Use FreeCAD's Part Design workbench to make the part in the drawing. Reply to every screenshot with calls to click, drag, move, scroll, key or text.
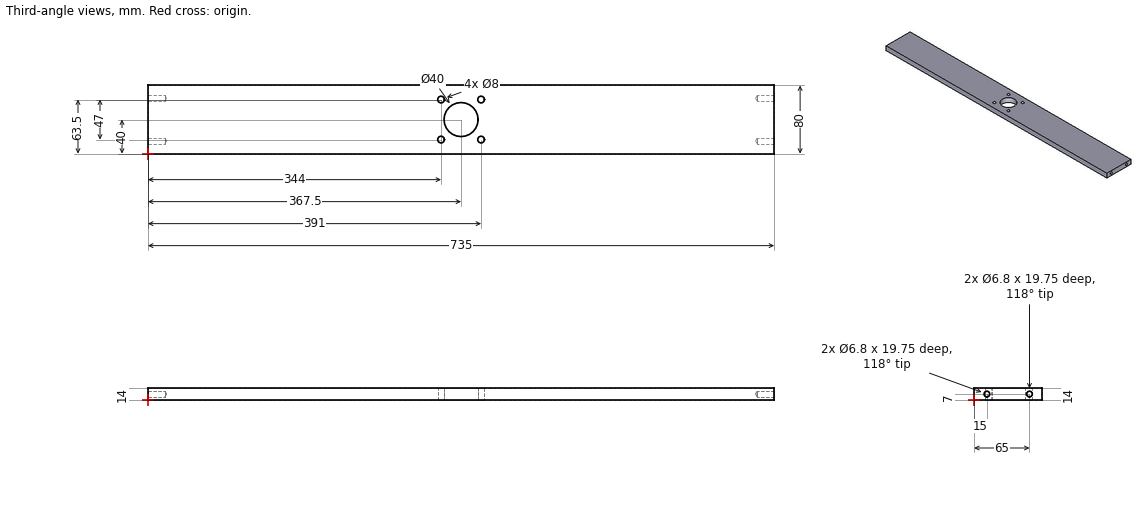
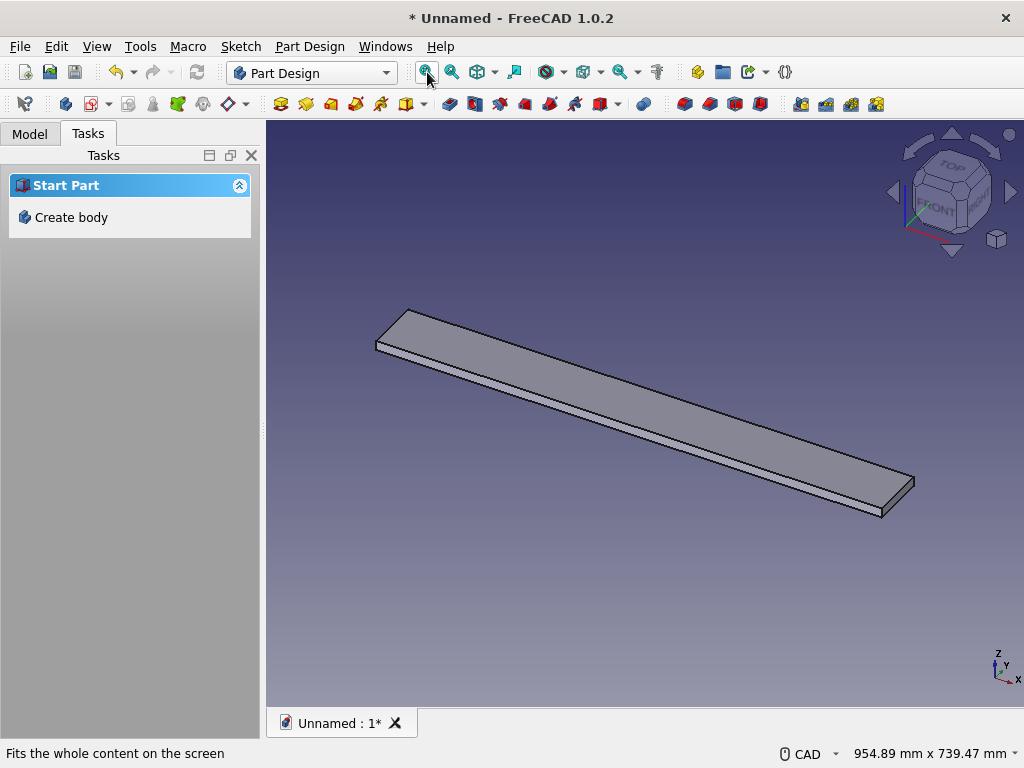
click(862, 480)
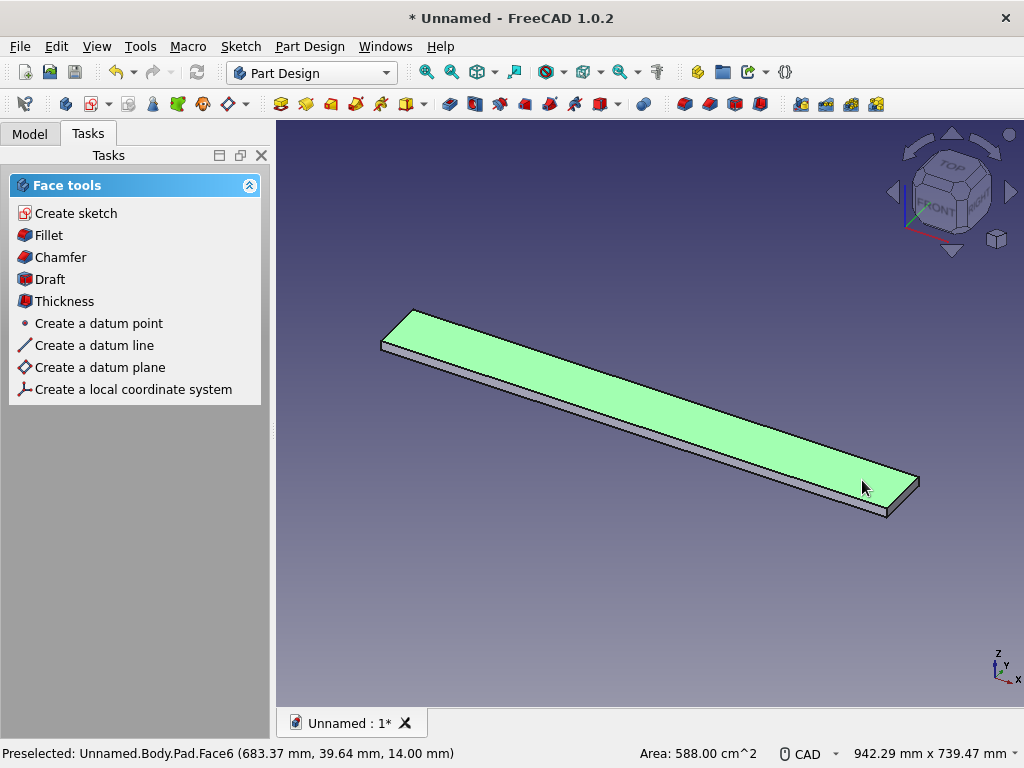
click(90, 104)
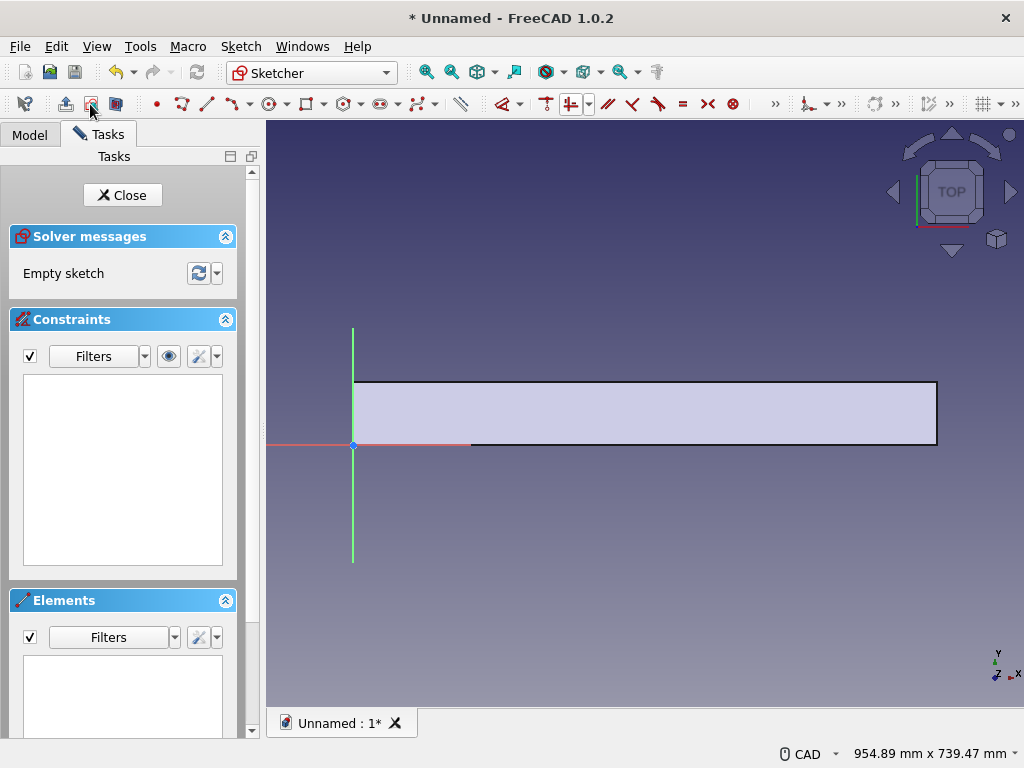
scroll(654, 414, up, 11)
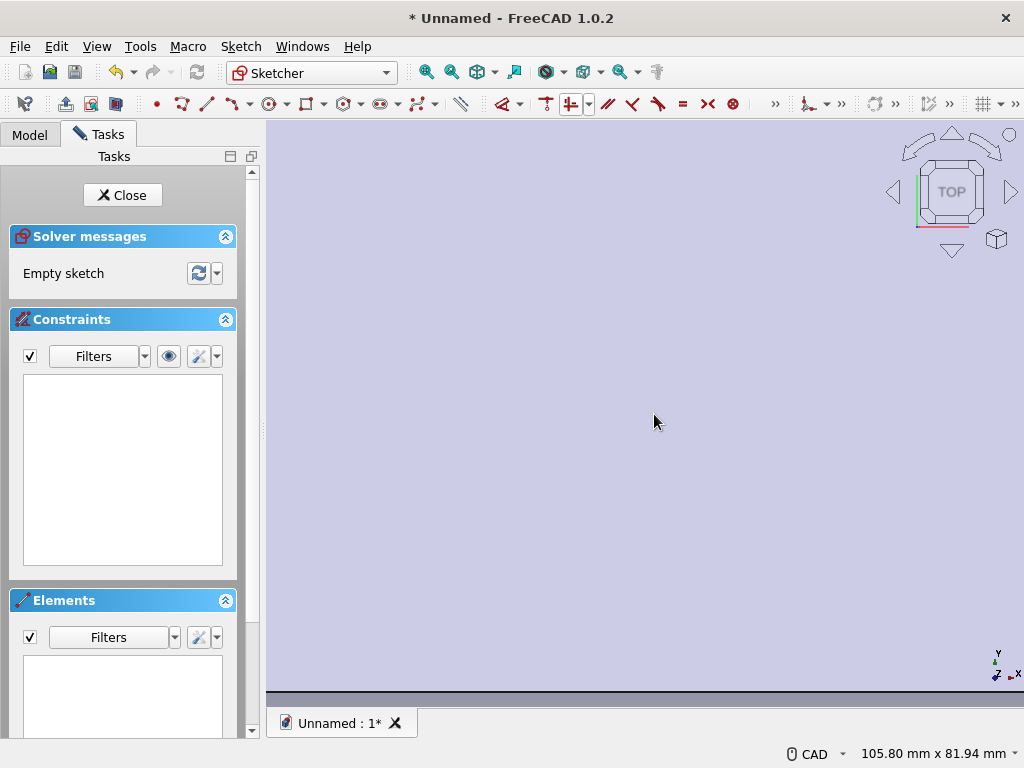
key(g)
key(c)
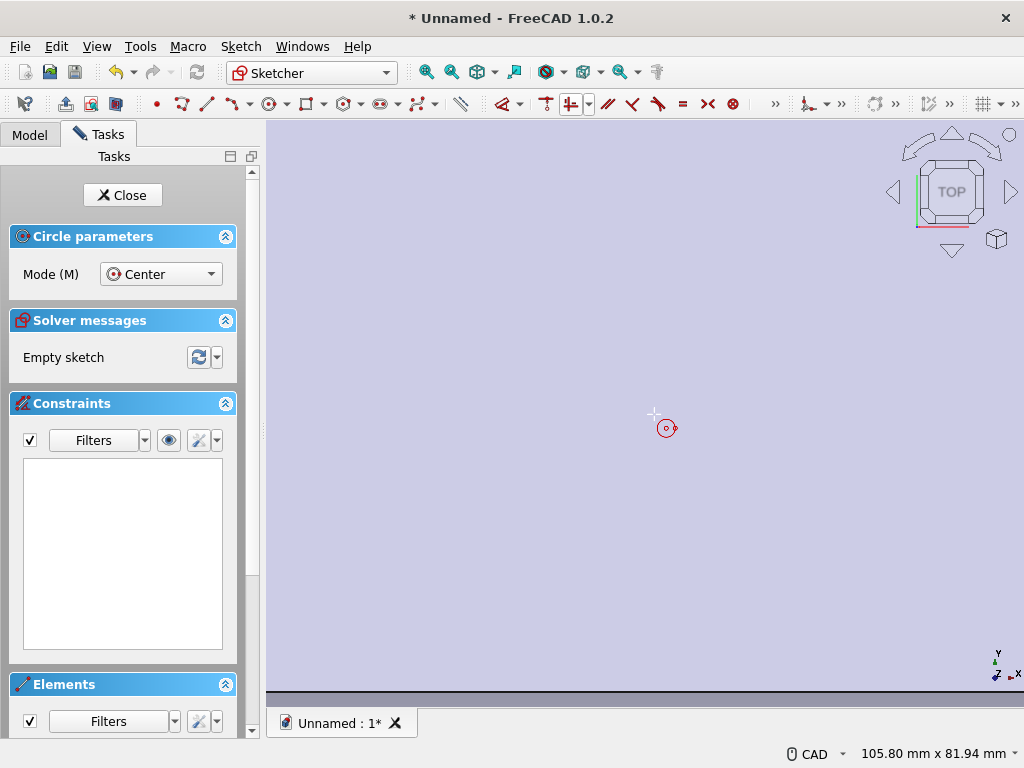
click(400, 237)
move(421, 217)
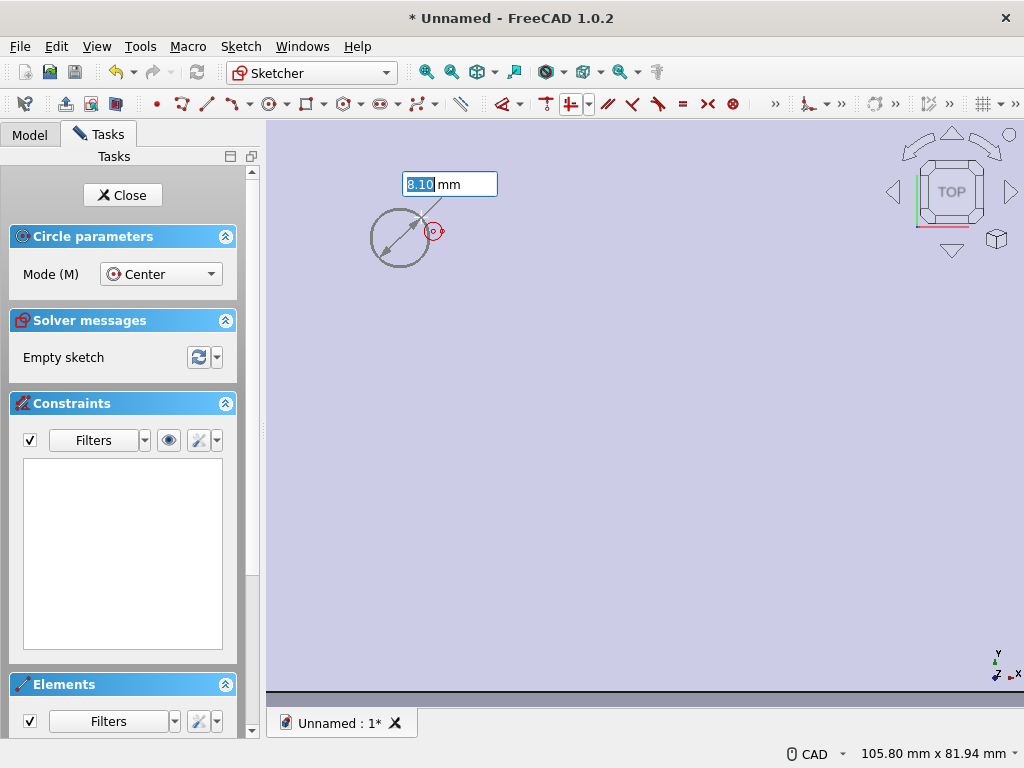
text(8)
key(Return)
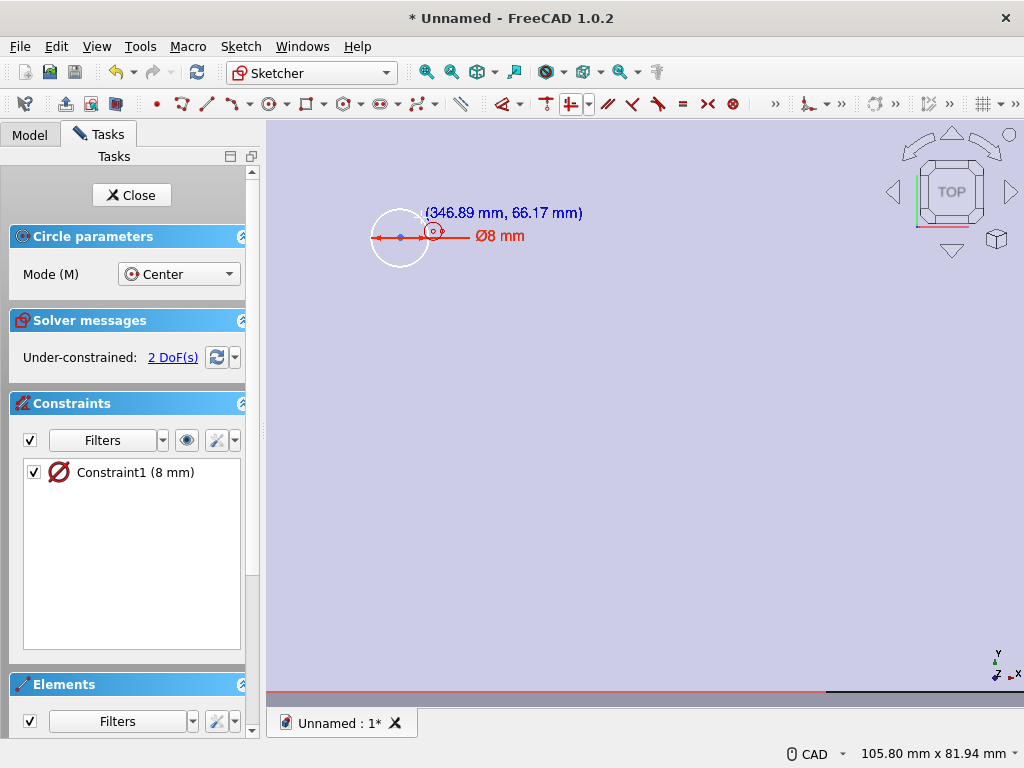
click(400, 574)
move(421, 554)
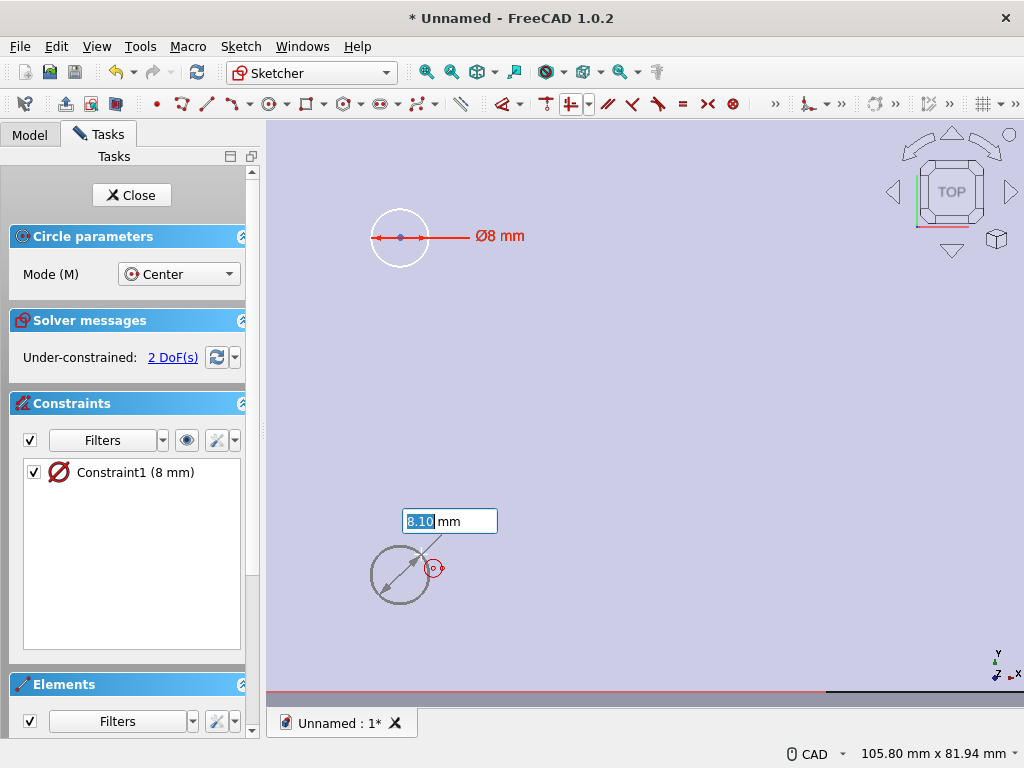
text(8)
key(Return)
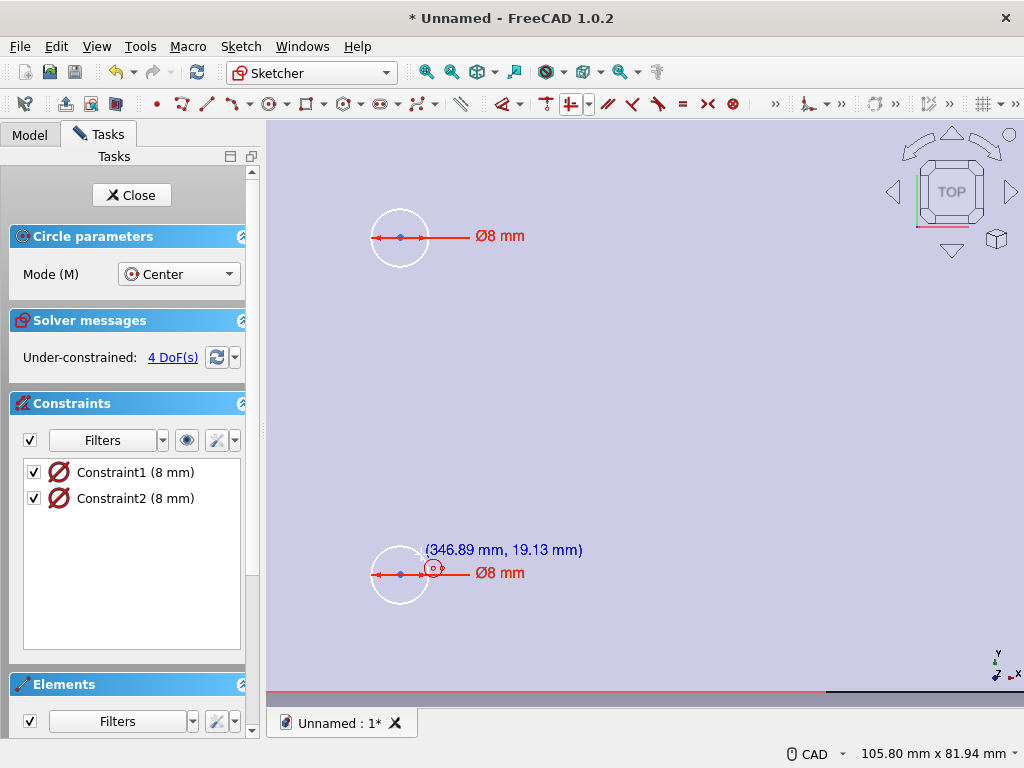
click(737, 574)
move(757, 554)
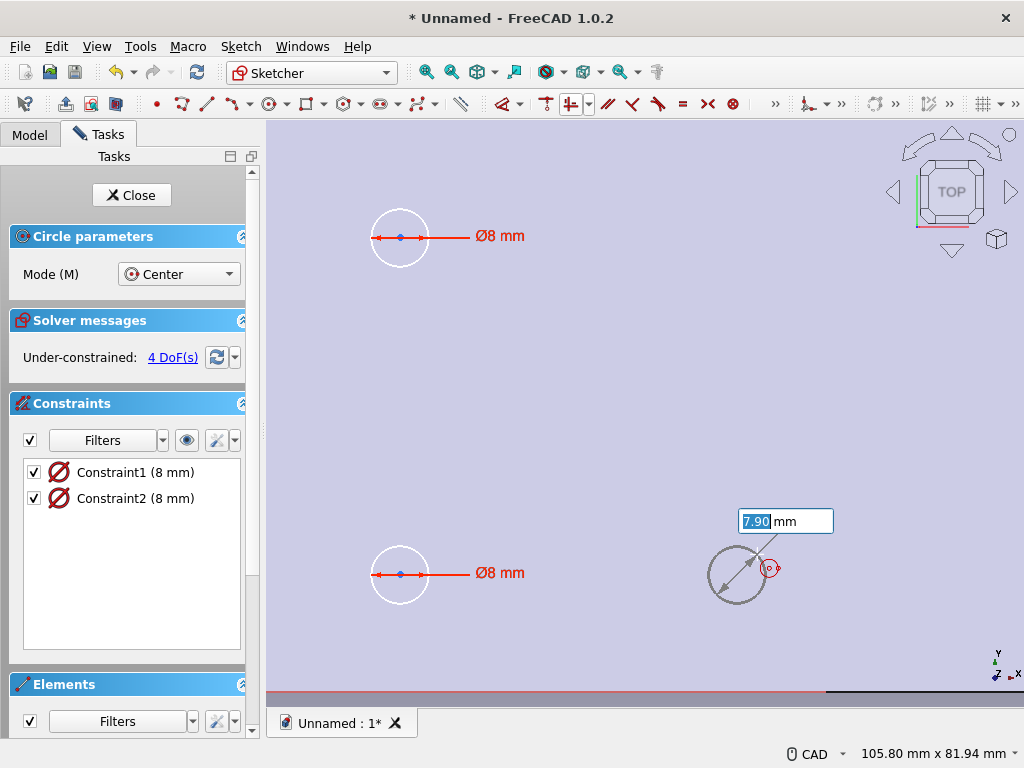
text(8)
key(Return)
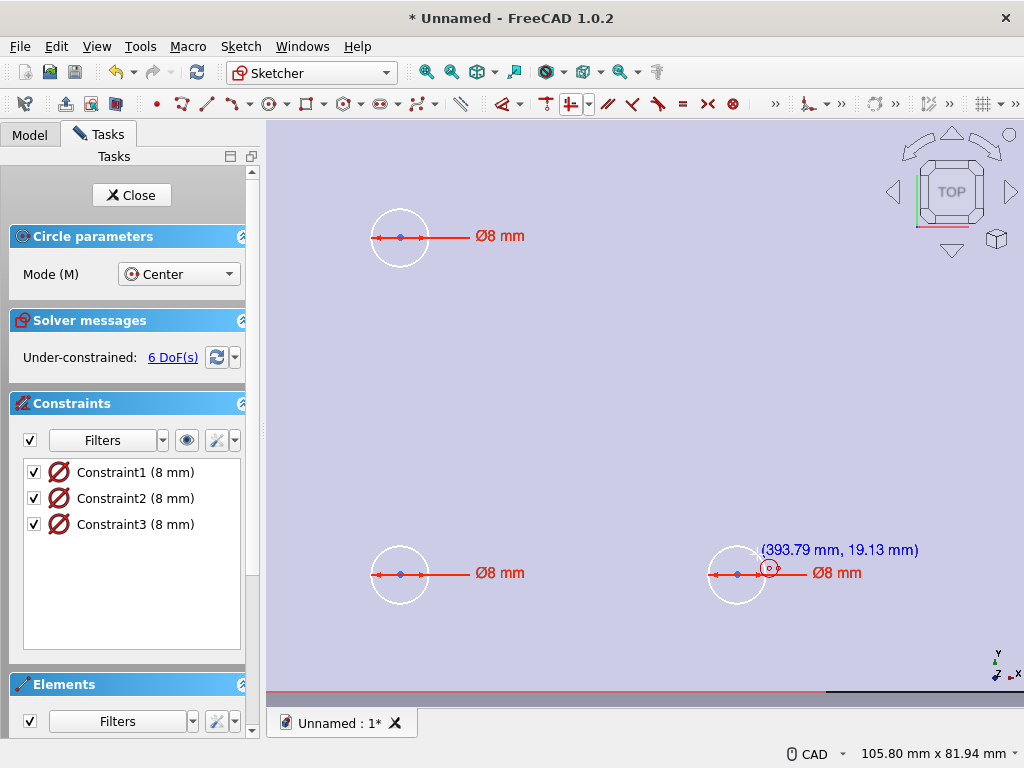
click(737, 237)
move(757, 217)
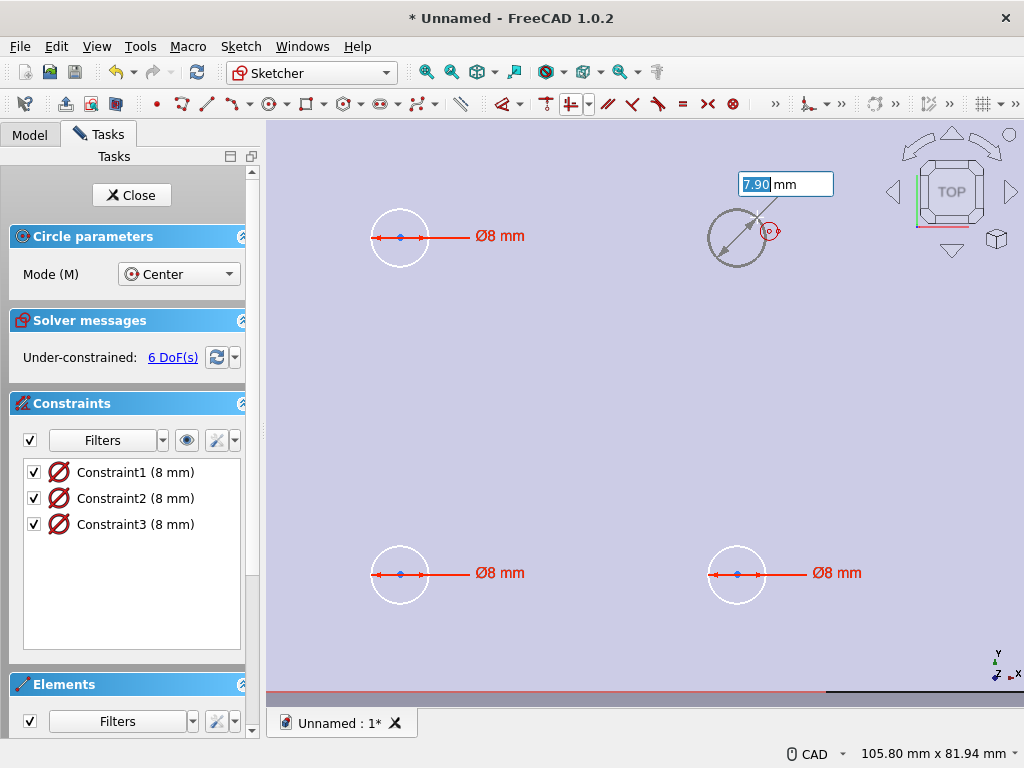
text(8)
key(Return)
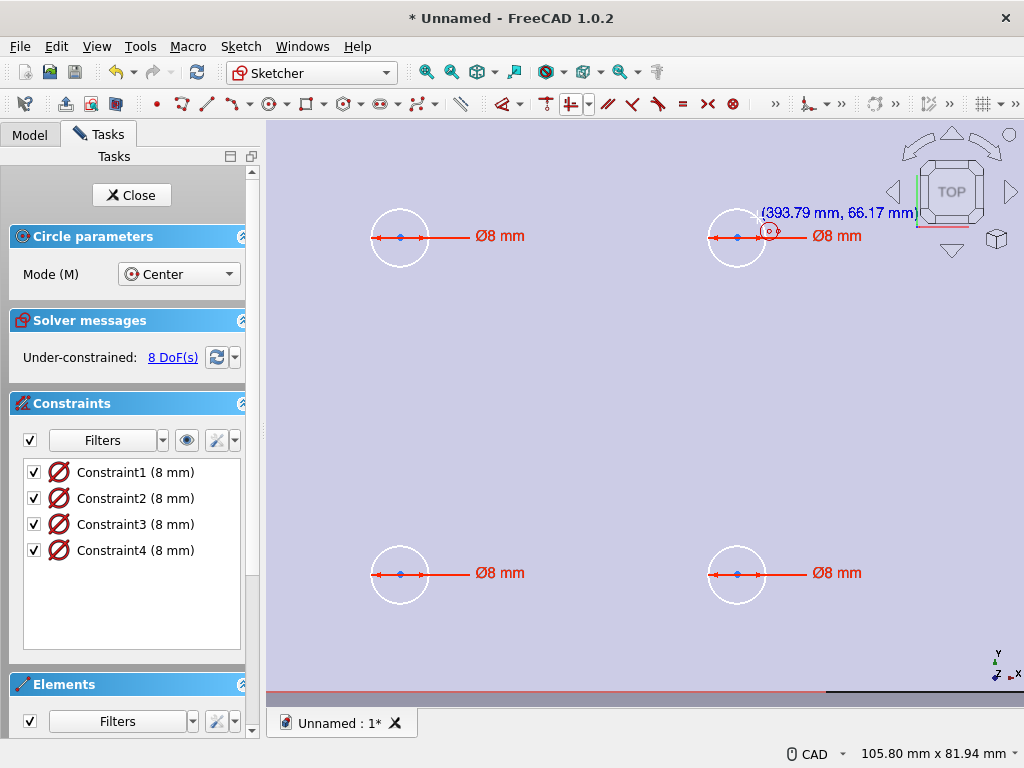
click(569, 405)
move(670, 304)